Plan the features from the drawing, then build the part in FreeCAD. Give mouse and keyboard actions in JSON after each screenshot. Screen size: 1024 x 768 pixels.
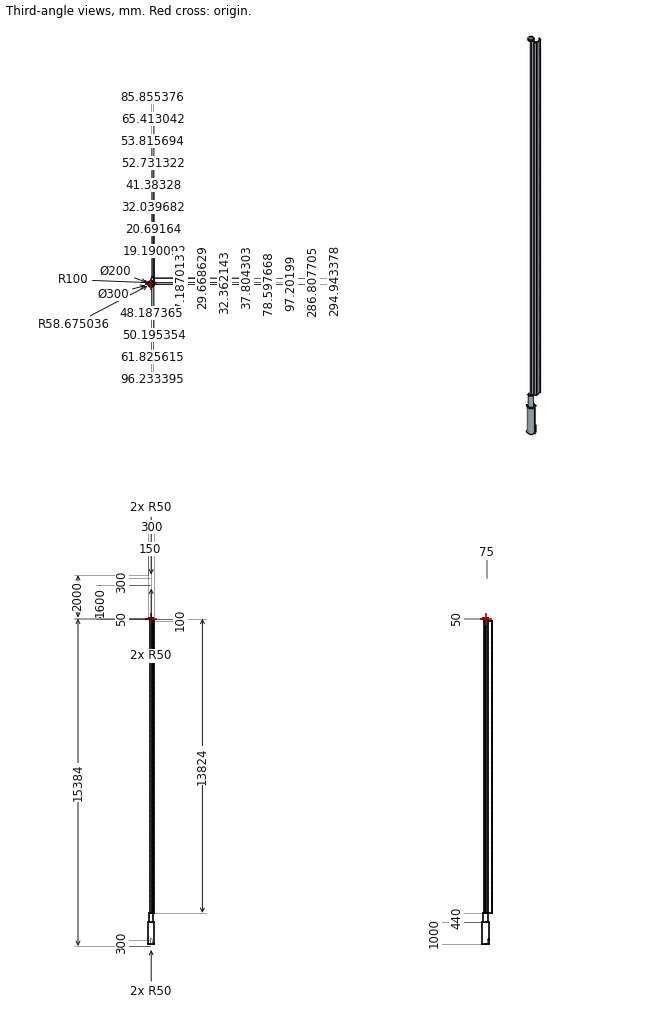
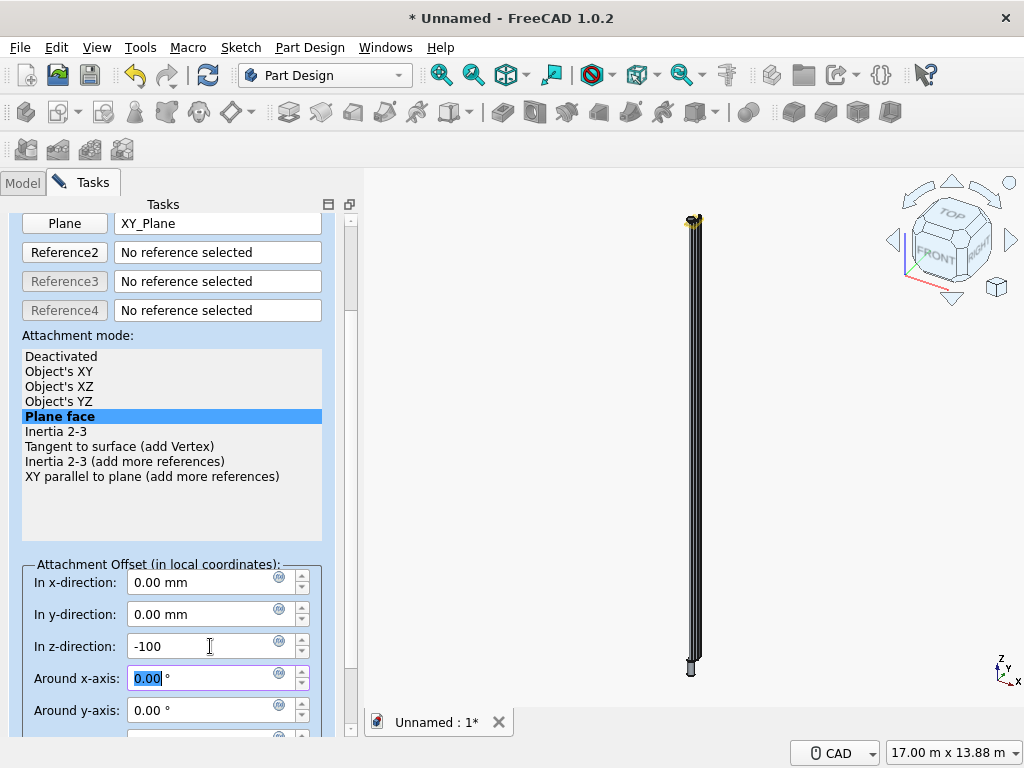
{"action": "scroll", "coordinate": [351, 475], "scroll_direction": "up", "scroll_amount": 3}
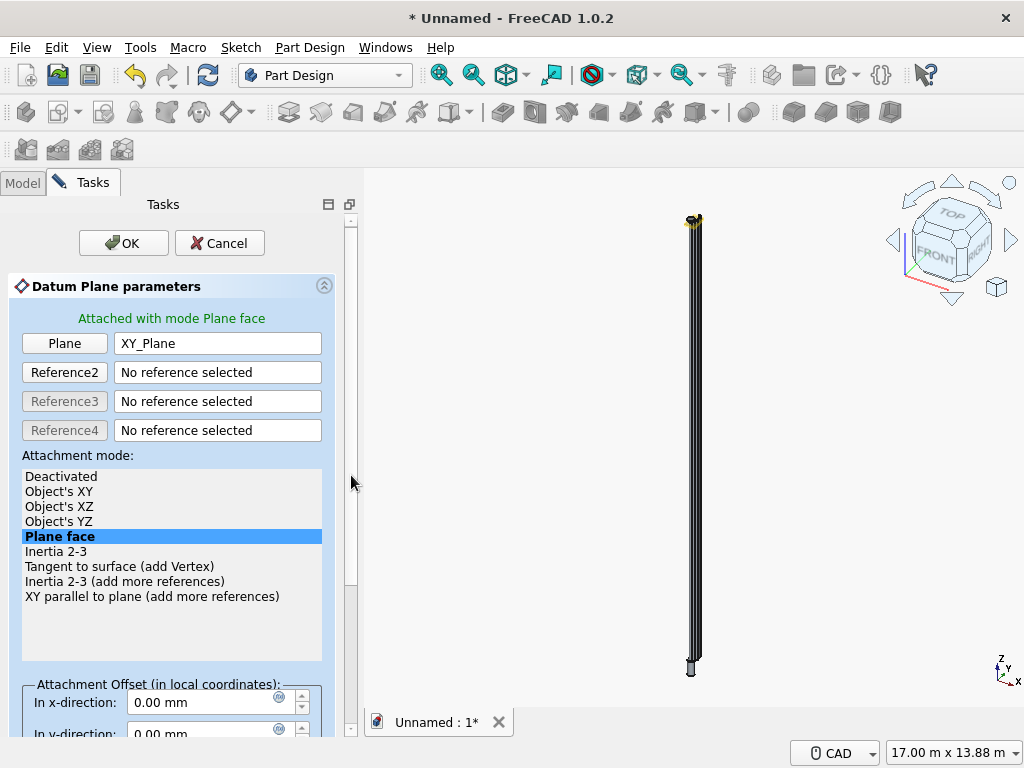
{"action": "left_click", "coordinate": [124, 243]}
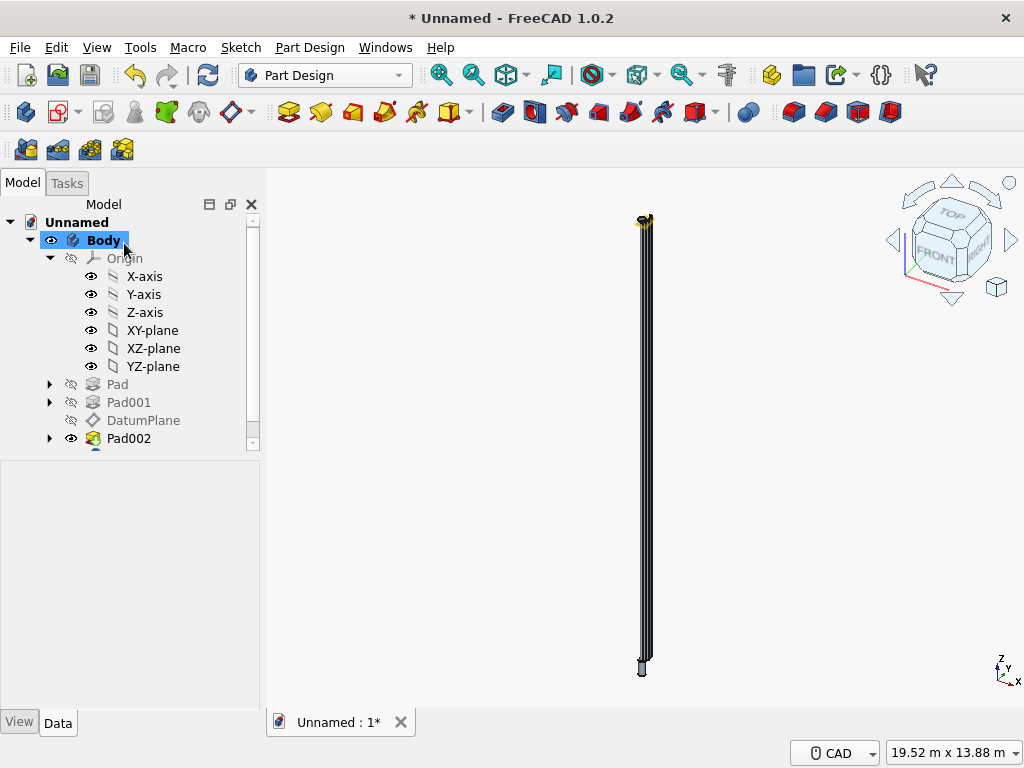
{"action": "scroll", "coordinate": [100, 326], "scroll_direction": "down", "scroll_amount": 3}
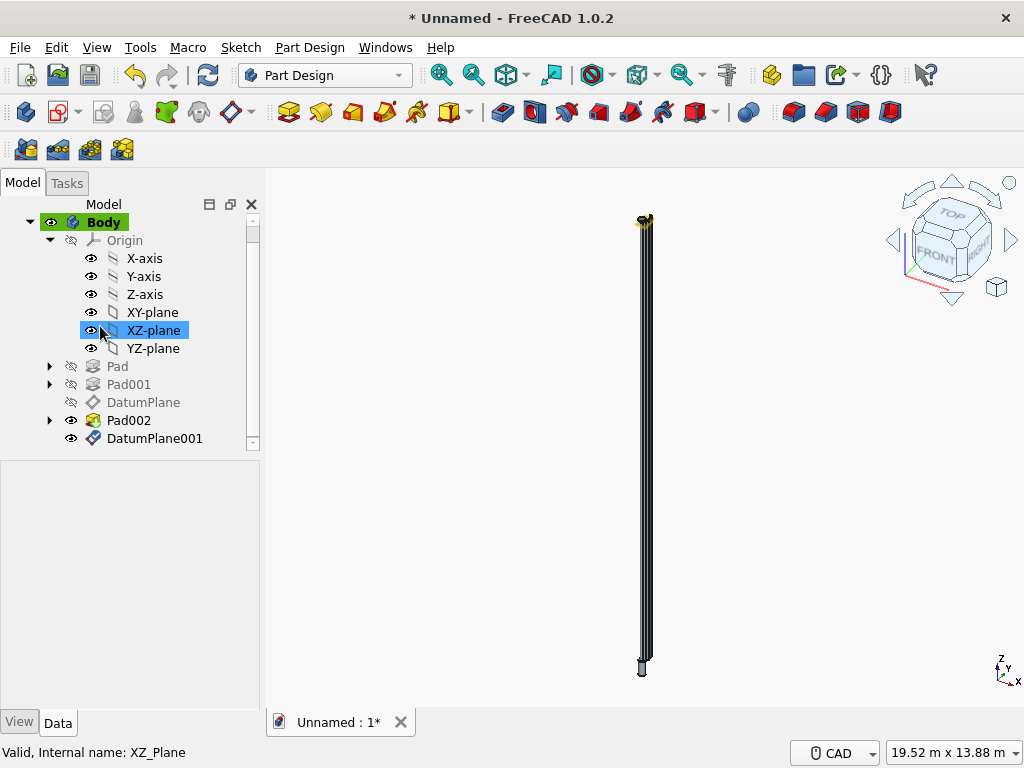
{"action": "left_click", "coordinate": [116, 438]}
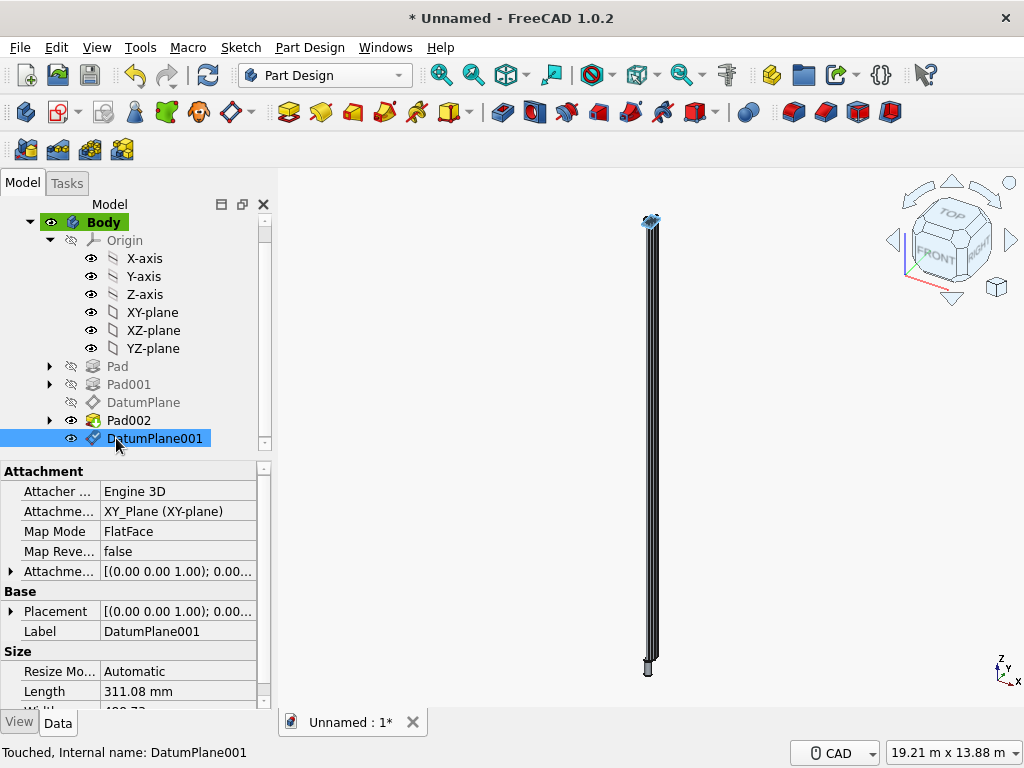
{"action": "left_click", "coordinate": [58, 112]}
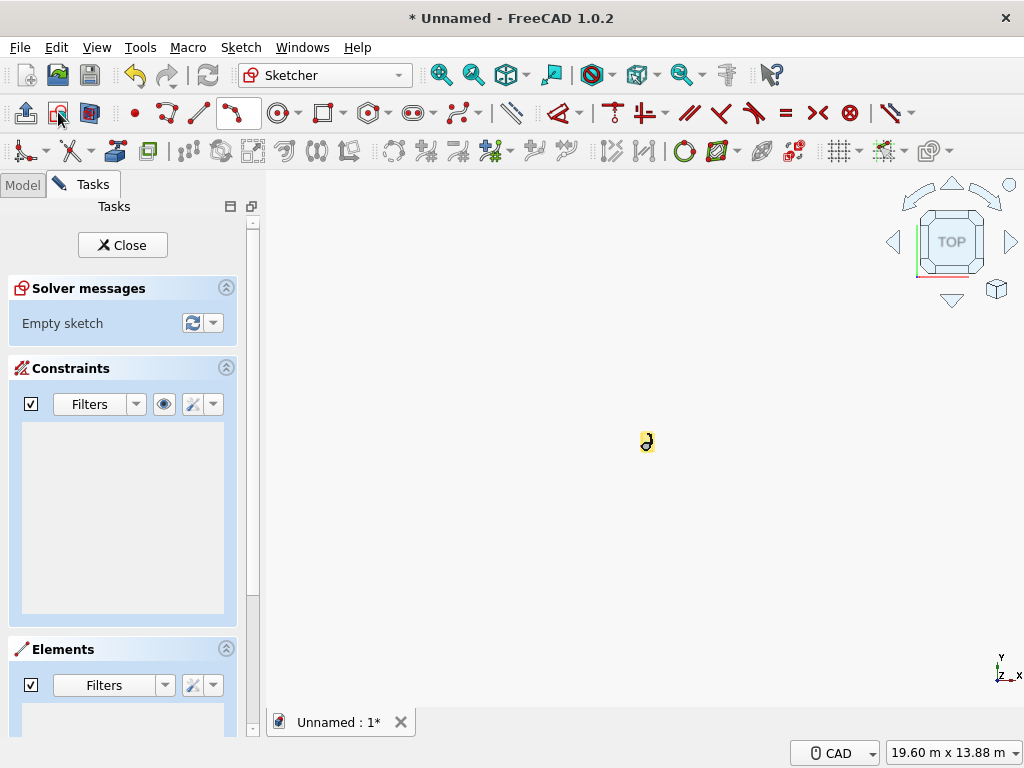
{"action": "left_click", "coordinate": [90, 114]}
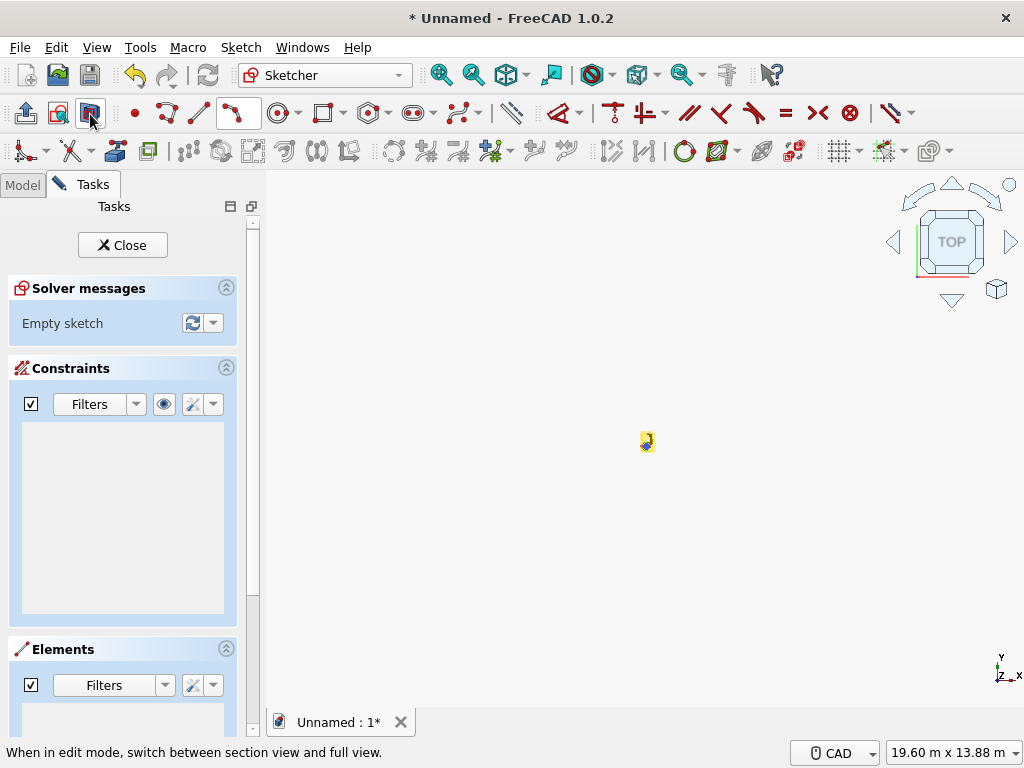
{"action": "scroll", "coordinate": [653, 440], "scroll_direction": "up", "scroll_amount": 15}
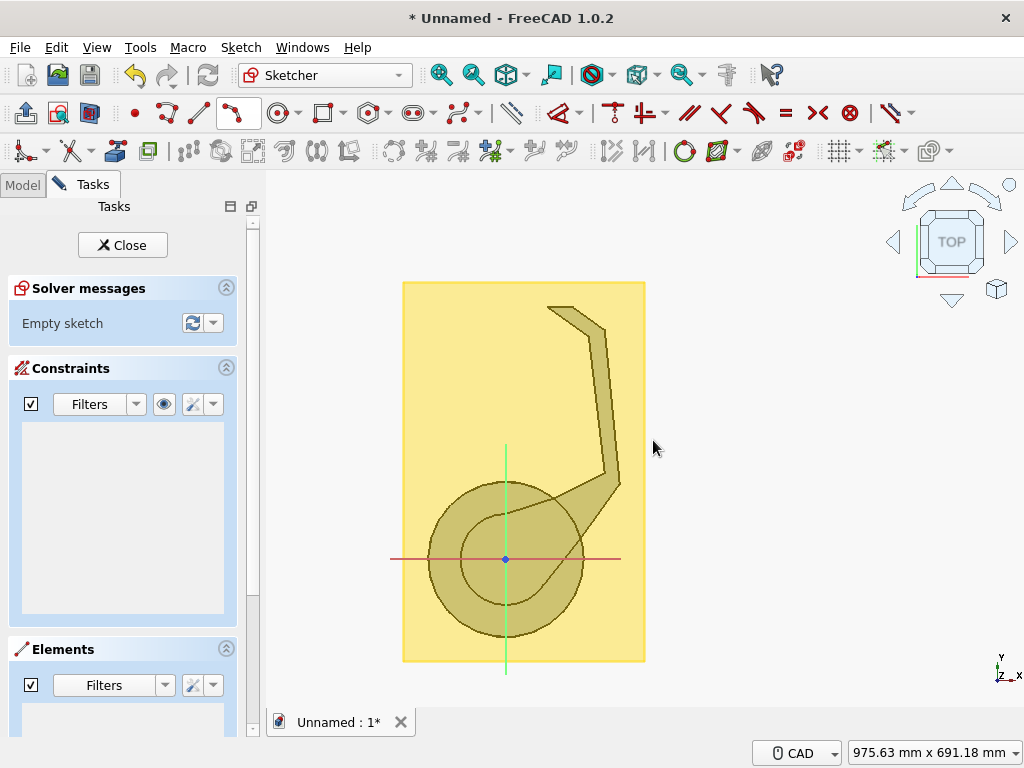
{"action": "left_click", "coordinate": [168, 114]}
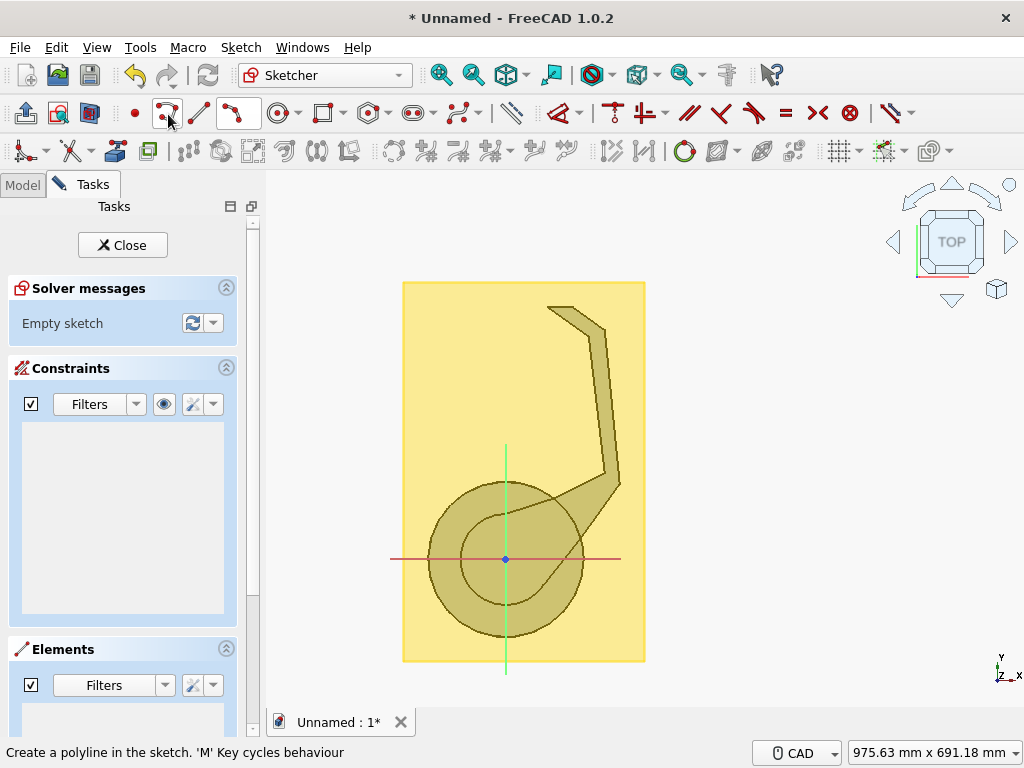
{"action": "left_click", "coordinate": [581, 538]}
{"action": "left_click", "coordinate": [620, 484]}
{"action": "left_click", "coordinate": [605, 330]}
{"action": "left_click", "coordinate": [573, 307]}
{"action": "left_click", "coordinate": [548, 307]}
{"action": "left_click", "coordinate": [589, 337]}
{"action": "left_click", "coordinate": [605, 473]}
{"action": "left_click", "coordinate": [554, 498]}
{"action": "right_click", "coordinate": [554, 498]}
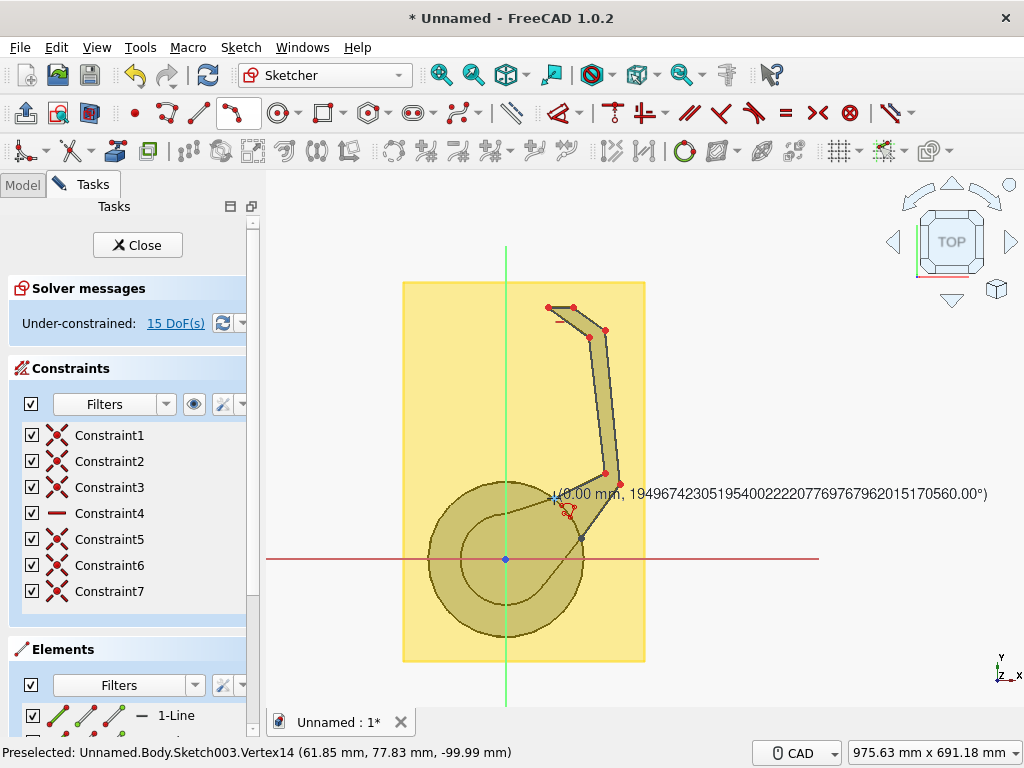
{"action": "left_click", "coordinate": [232, 114]}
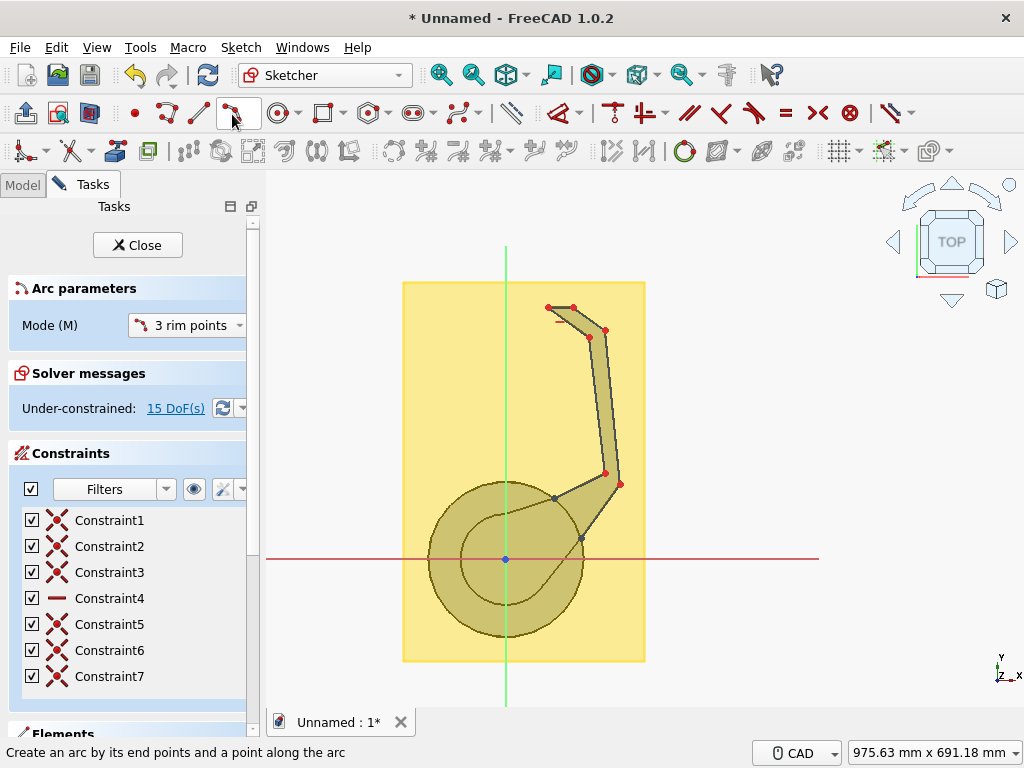
{"action": "left_click", "coordinate": [554, 499]}
{"action": "left_click", "coordinate": [581, 539]}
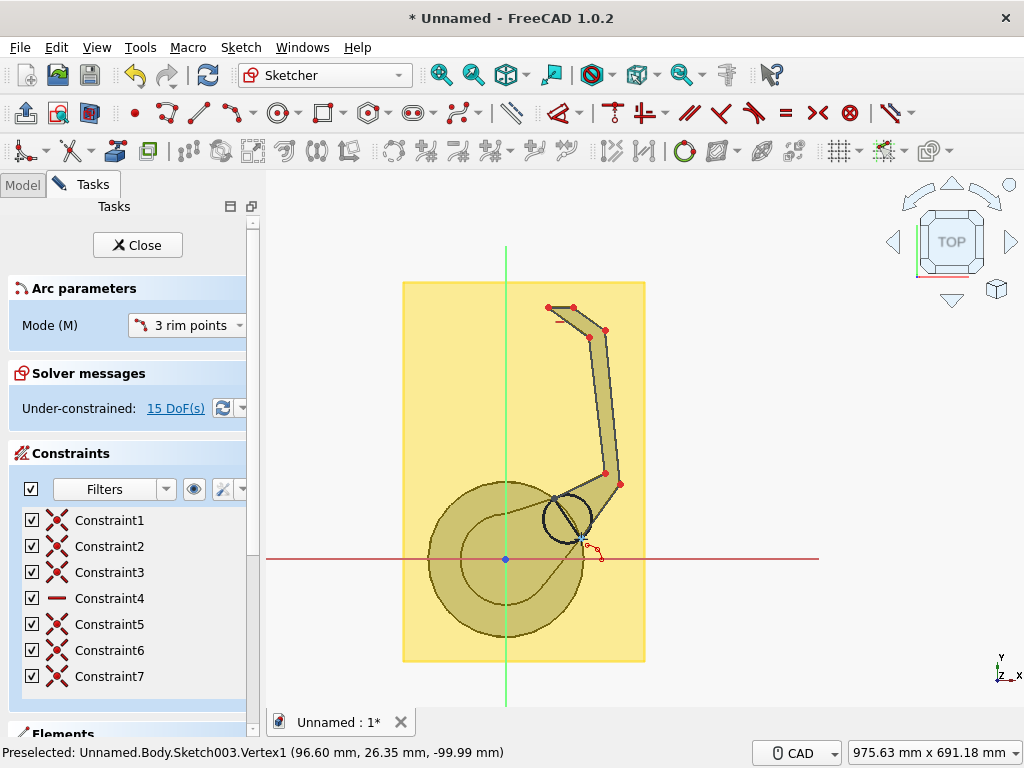
{"action": "scroll", "coordinate": [571, 516], "scroll_direction": "up", "scroll_amount": 8}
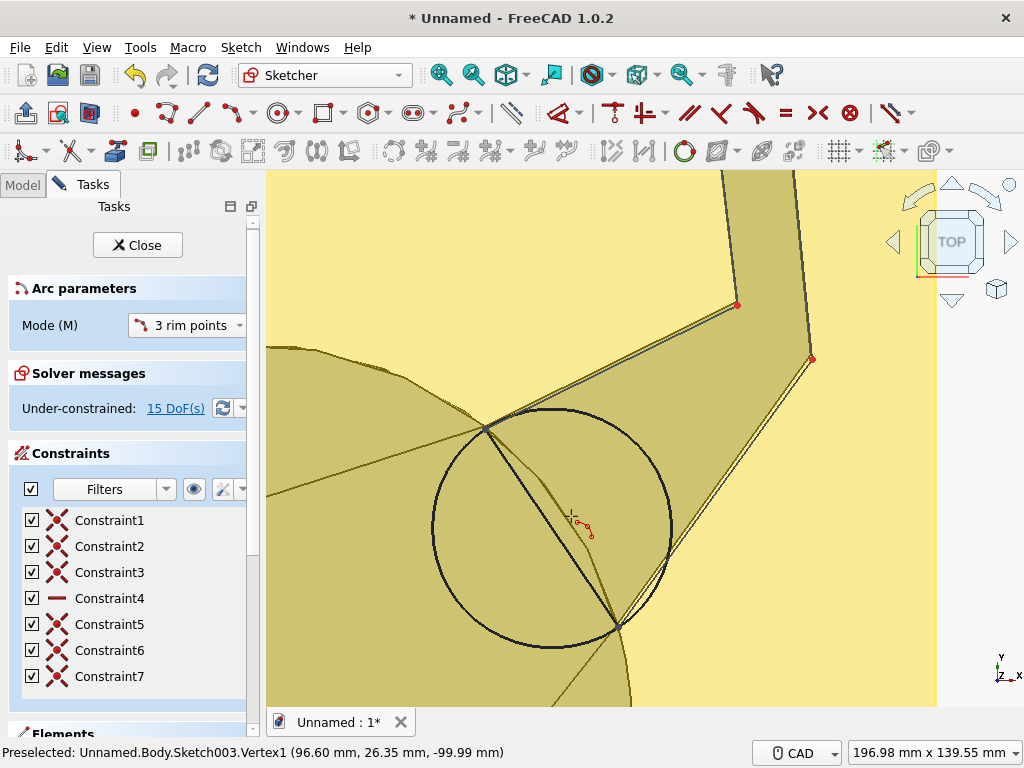
{"action": "left_click", "coordinate": [567, 515]}
{"action": "key", "text": "Escape"}